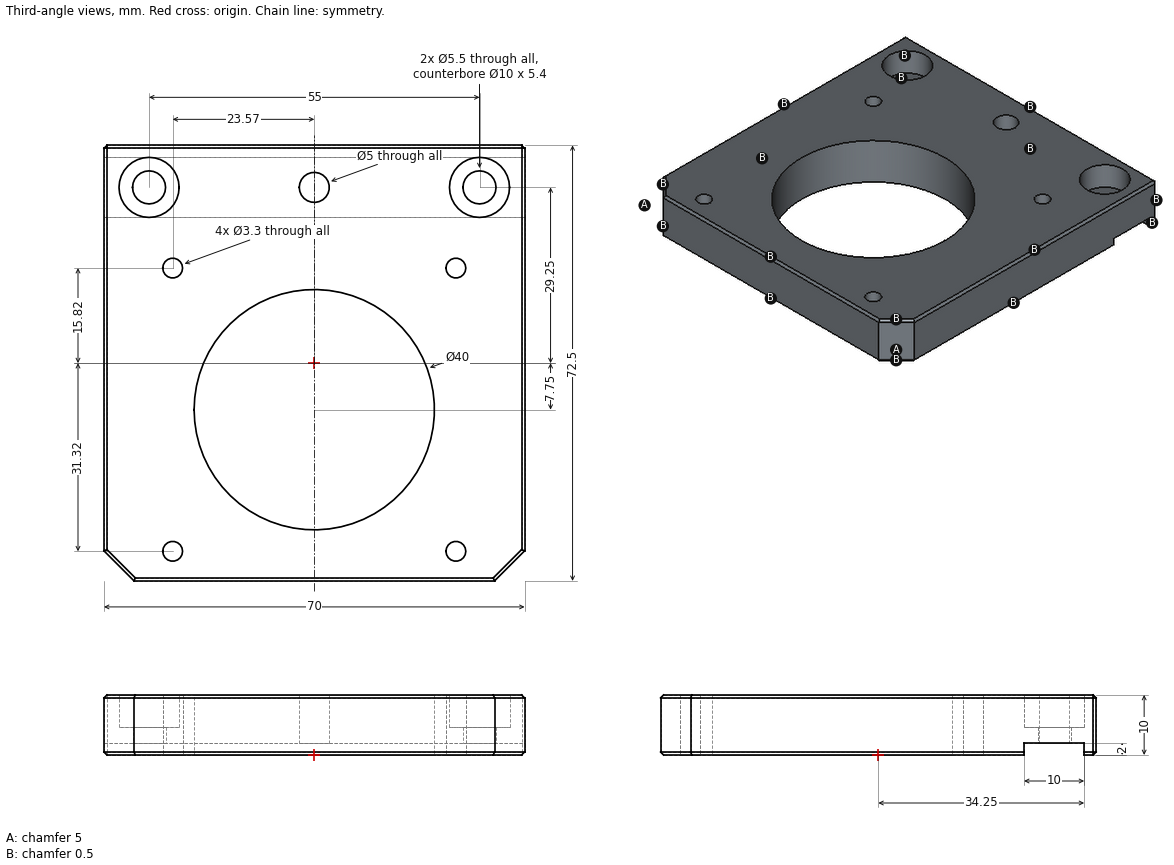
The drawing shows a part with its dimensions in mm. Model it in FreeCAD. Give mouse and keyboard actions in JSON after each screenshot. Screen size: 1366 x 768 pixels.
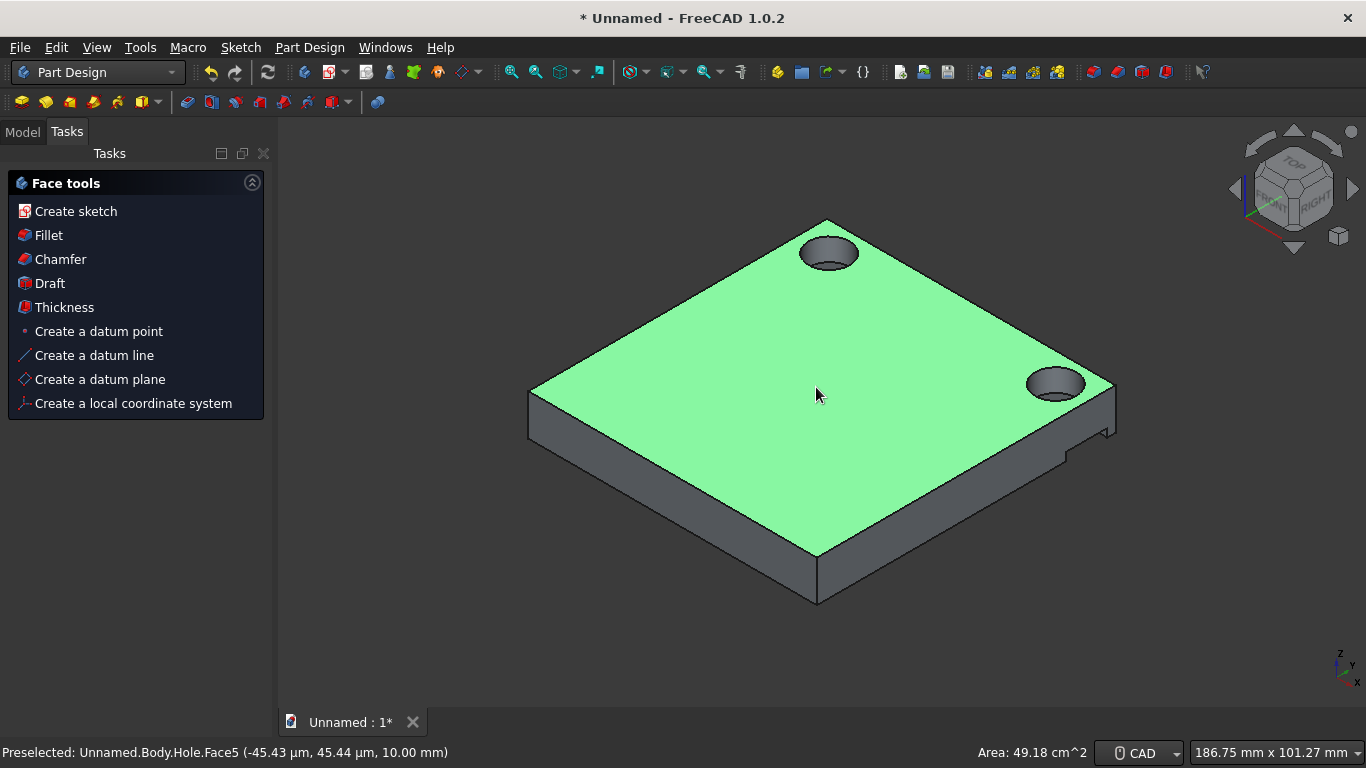
{"action": "left_click", "coordinate": [330, 72]}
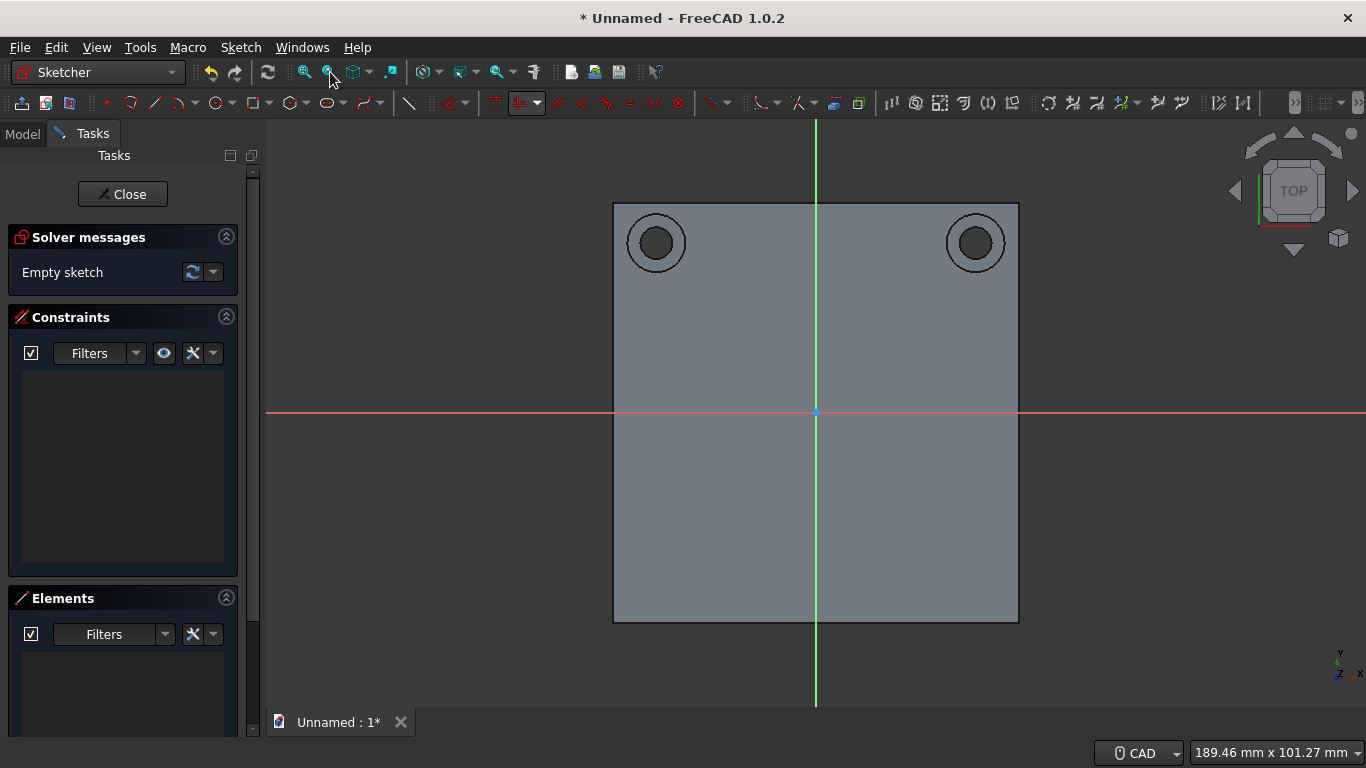
{"action": "scroll", "coordinate": [821, 230], "scroll_direction": "up", "scroll_amount": 13}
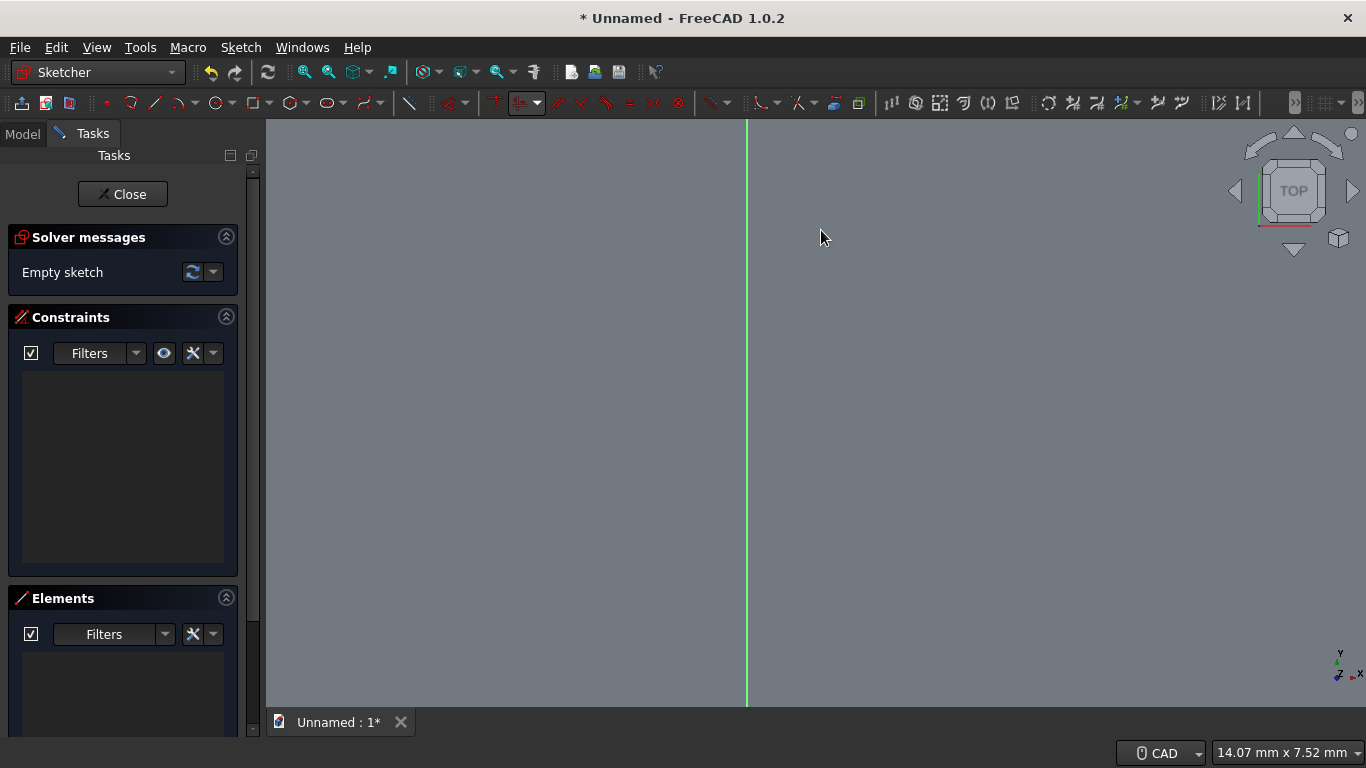
{"action": "left_click", "coordinate": [216, 104]}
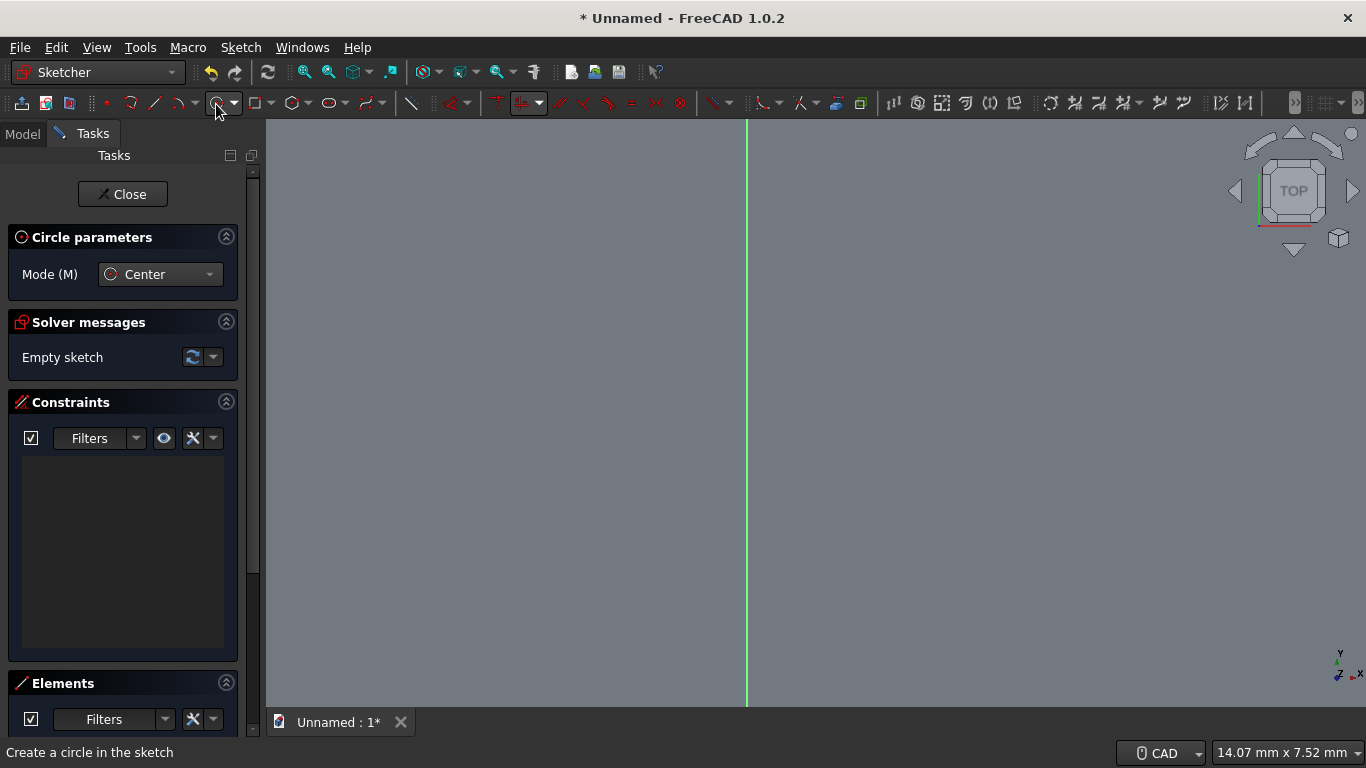
{"action": "left_click", "coordinate": [747, 405]}
{"action": "mouse_move", "coordinate": [886, 267]}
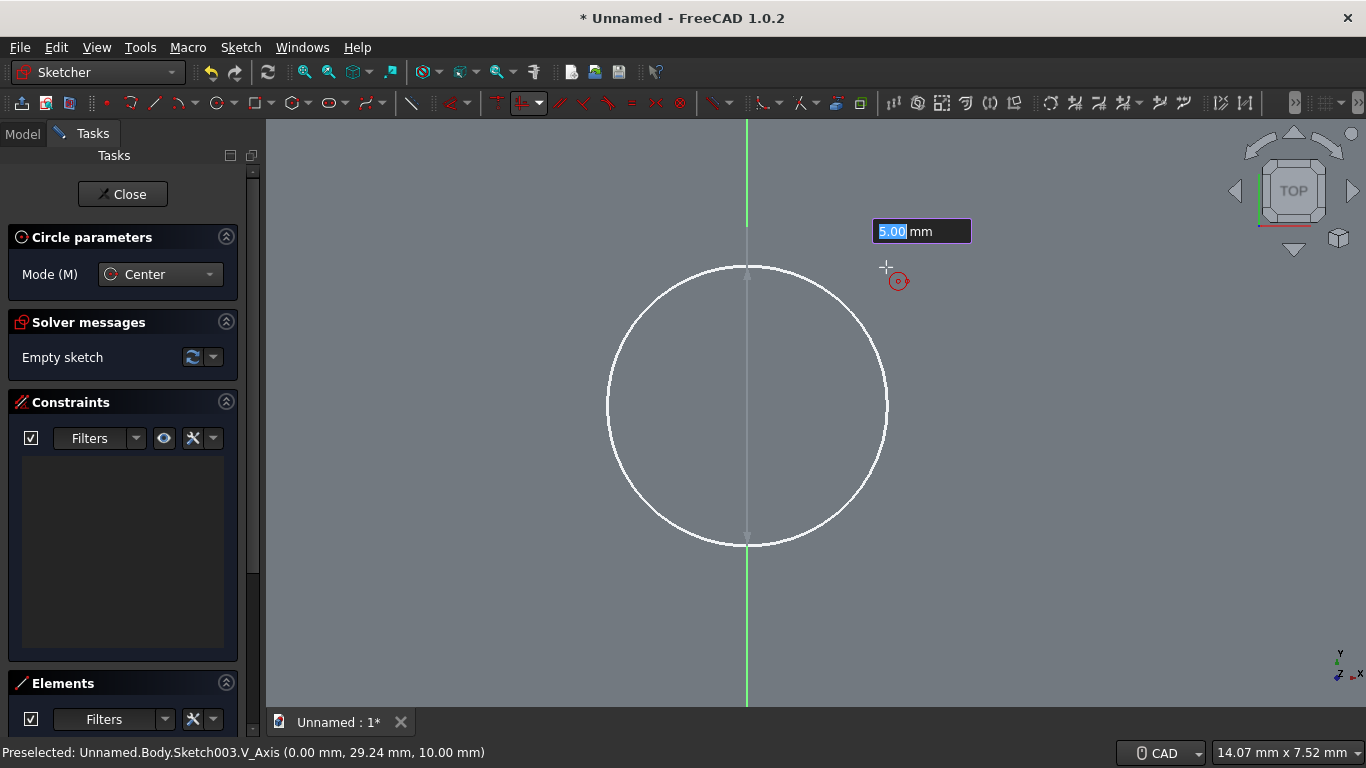
{"action": "type", "text": "5"}
{"action": "key", "text": "Return"}
{"action": "key", "text": "Escape"}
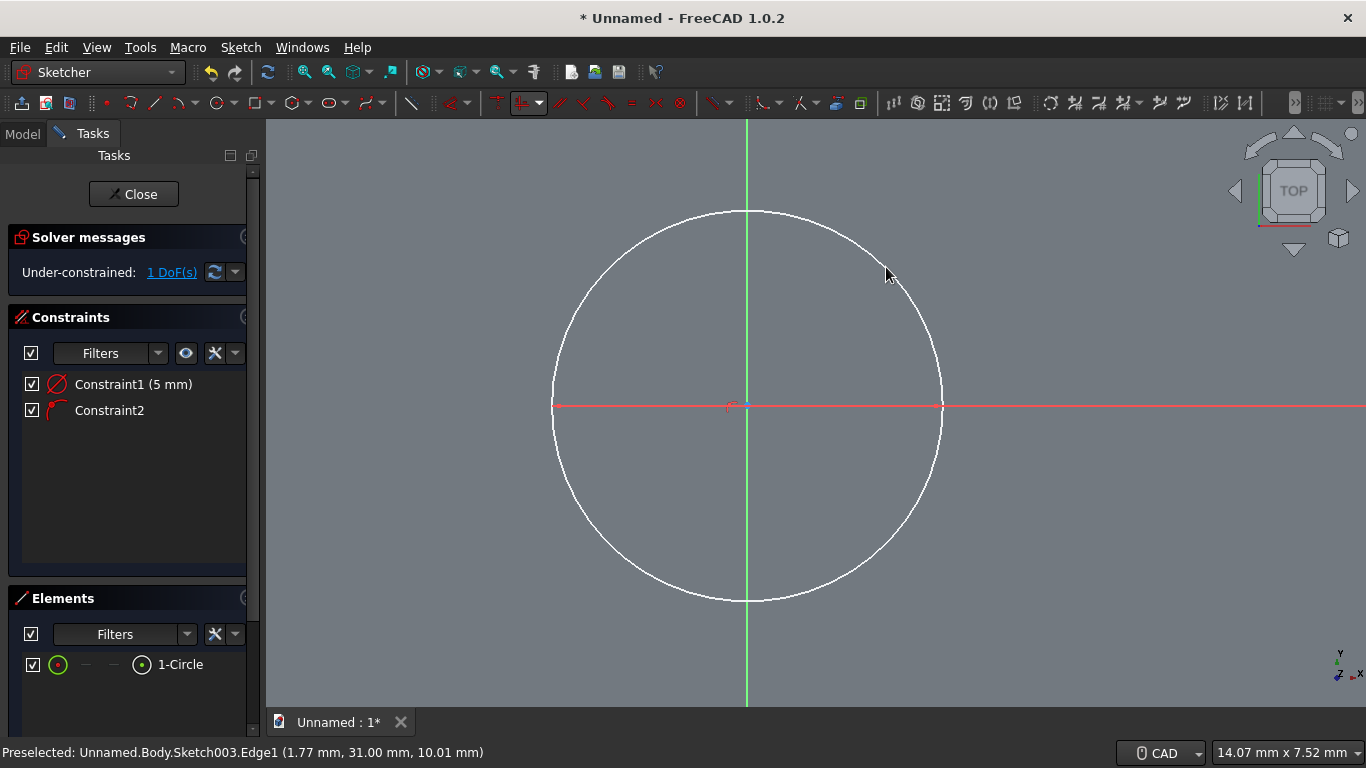
{"action": "left_click", "coordinate": [450, 104]}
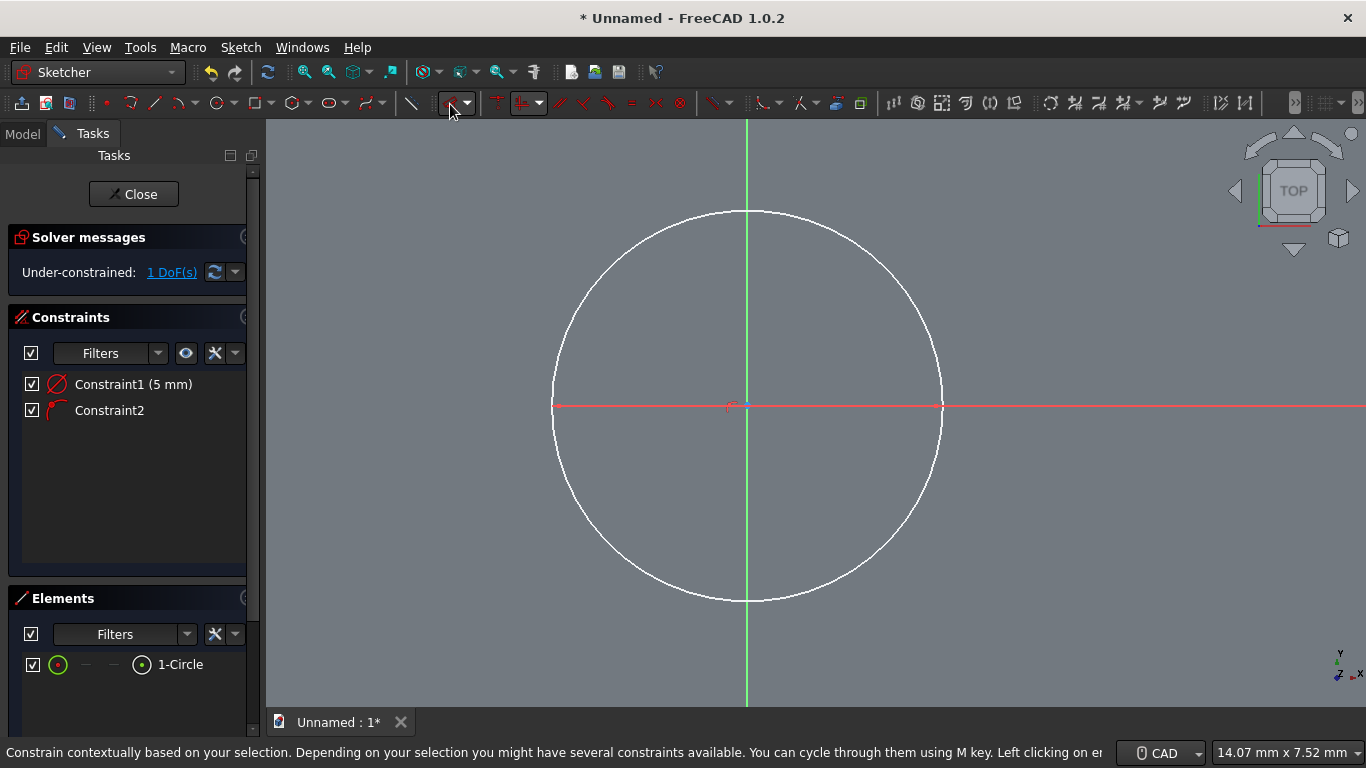
{"action": "left_click", "coordinate": [747, 406]}
{"action": "left_click", "coordinate": [781, 543]}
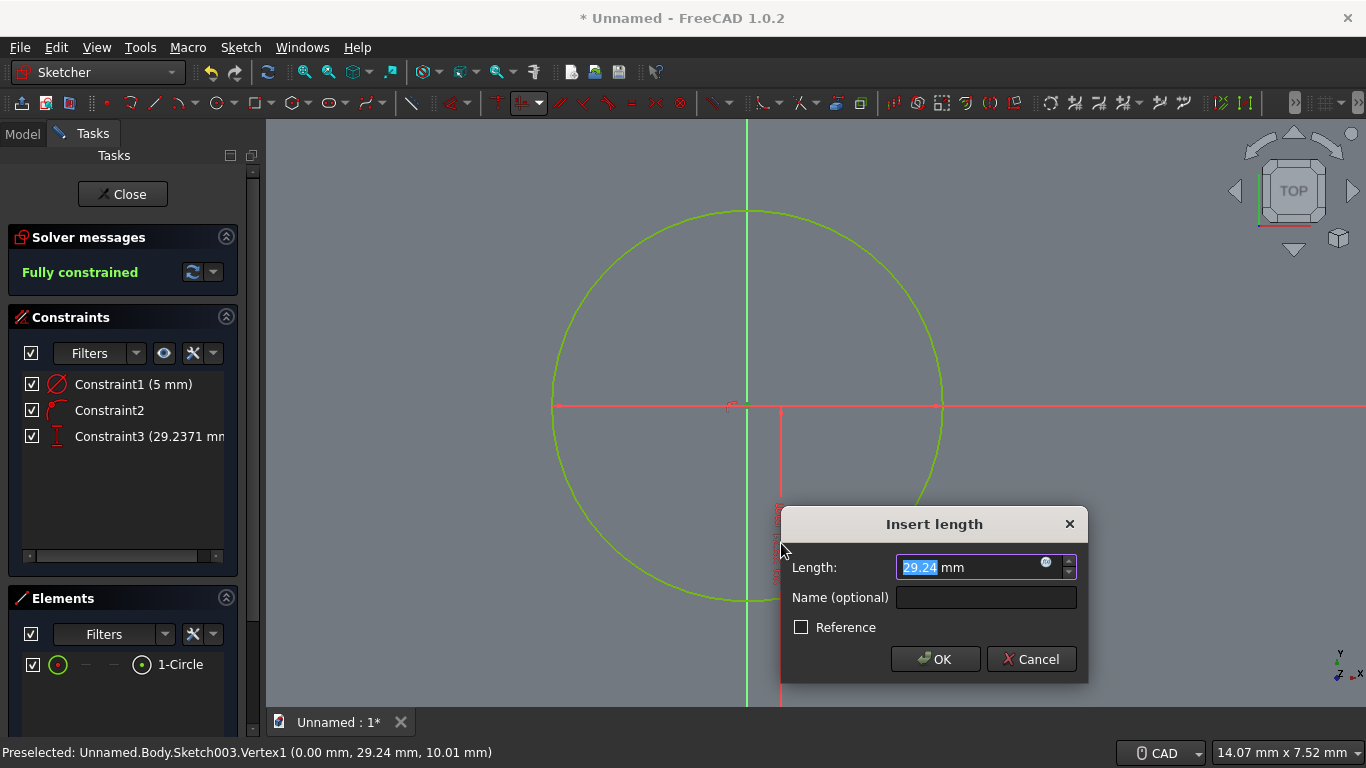
{"action": "type", "text": "29.25"}
{"action": "key", "text": "Return"}
{"action": "key", "text": "Escape"}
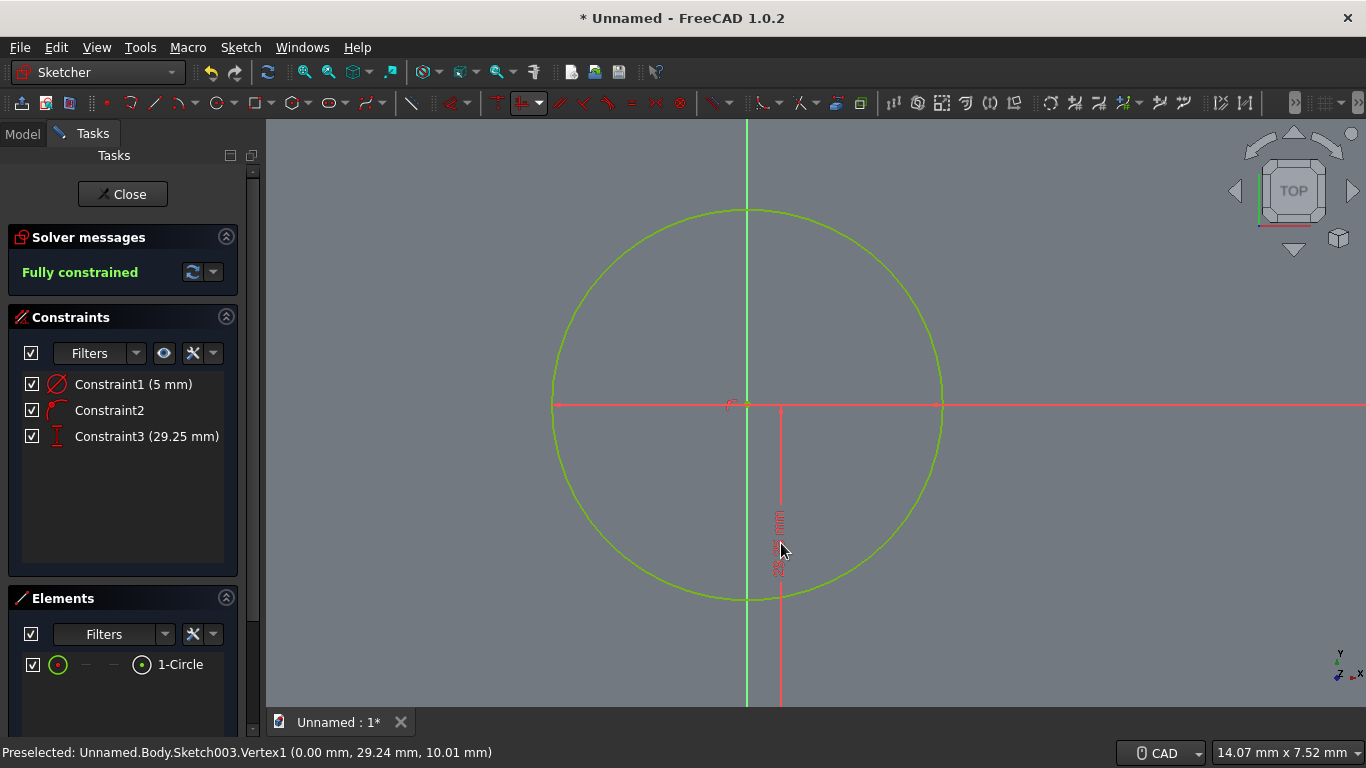
{"action": "left_click", "coordinate": [123, 194]}